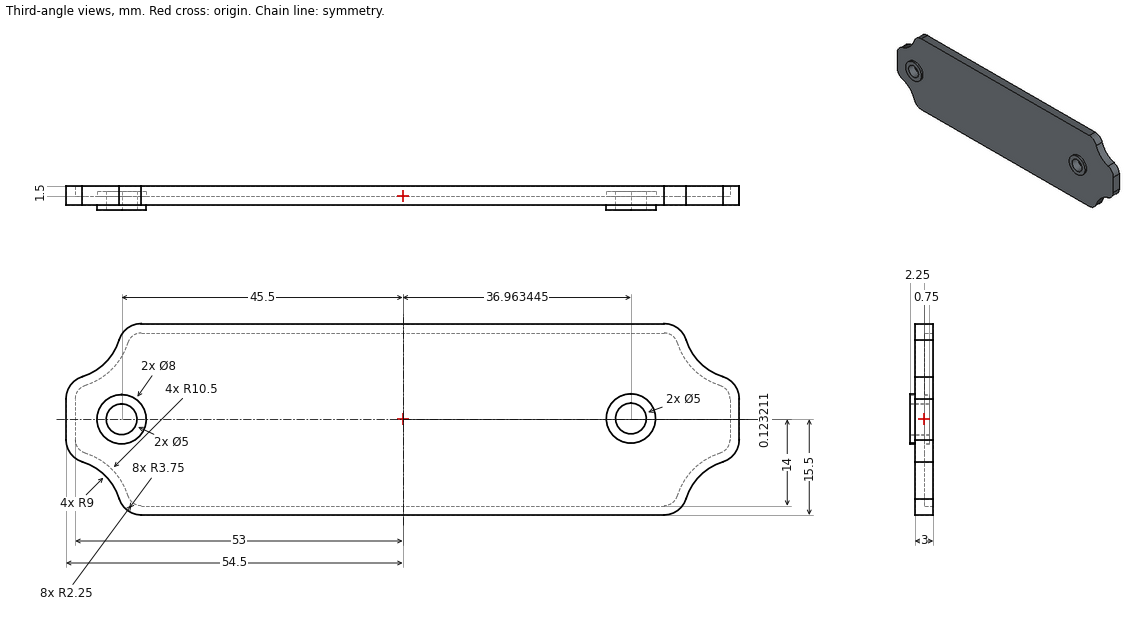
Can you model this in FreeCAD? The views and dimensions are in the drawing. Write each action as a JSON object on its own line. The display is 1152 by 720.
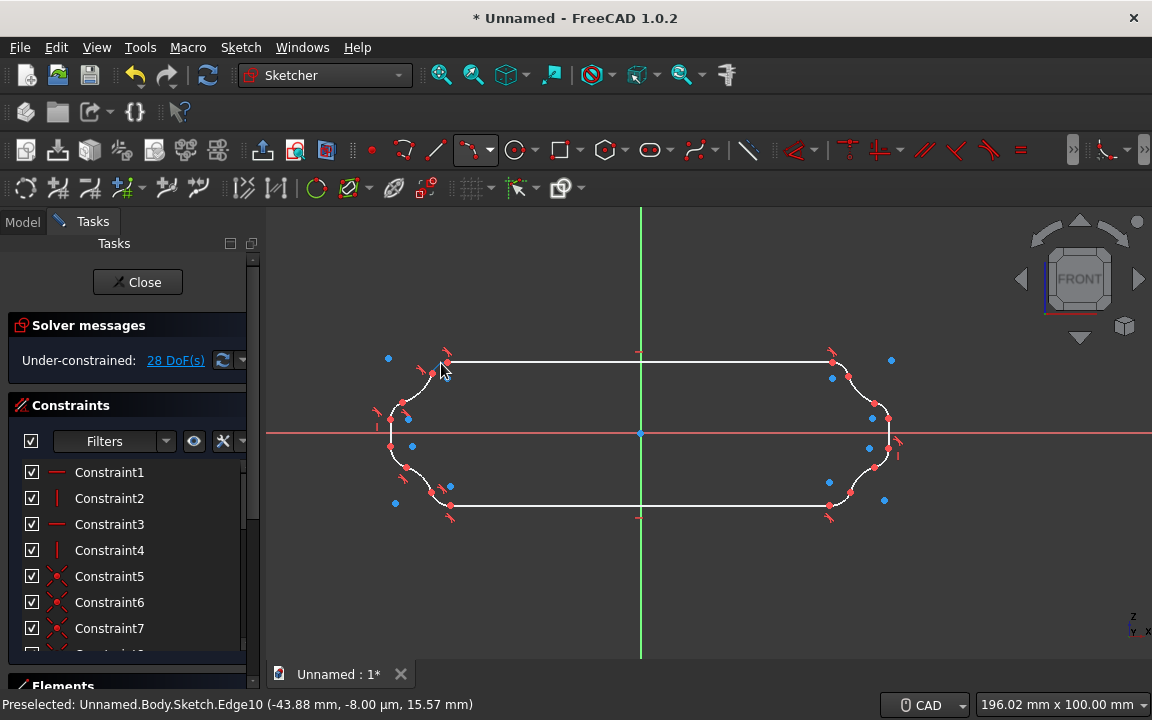
{"action": "scroll", "coordinate": [846, 370], "scroll_direction": "up", "scroll_amount": 4}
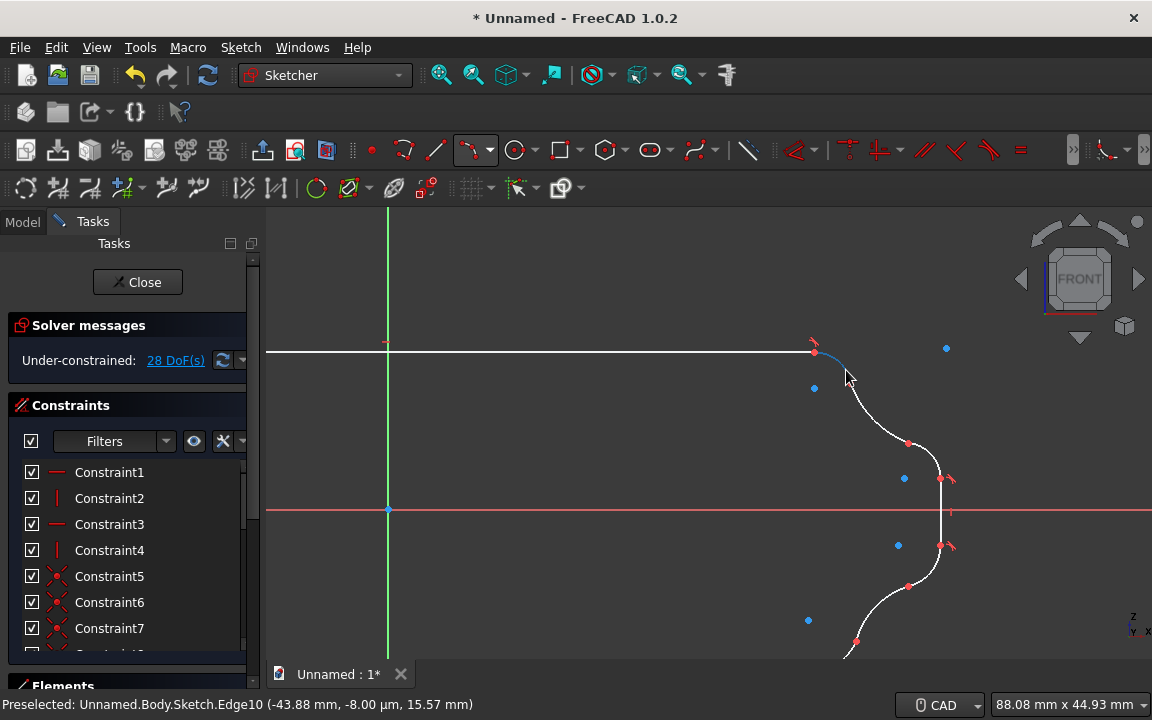
{"action": "left_click", "coordinate": [845, 369]}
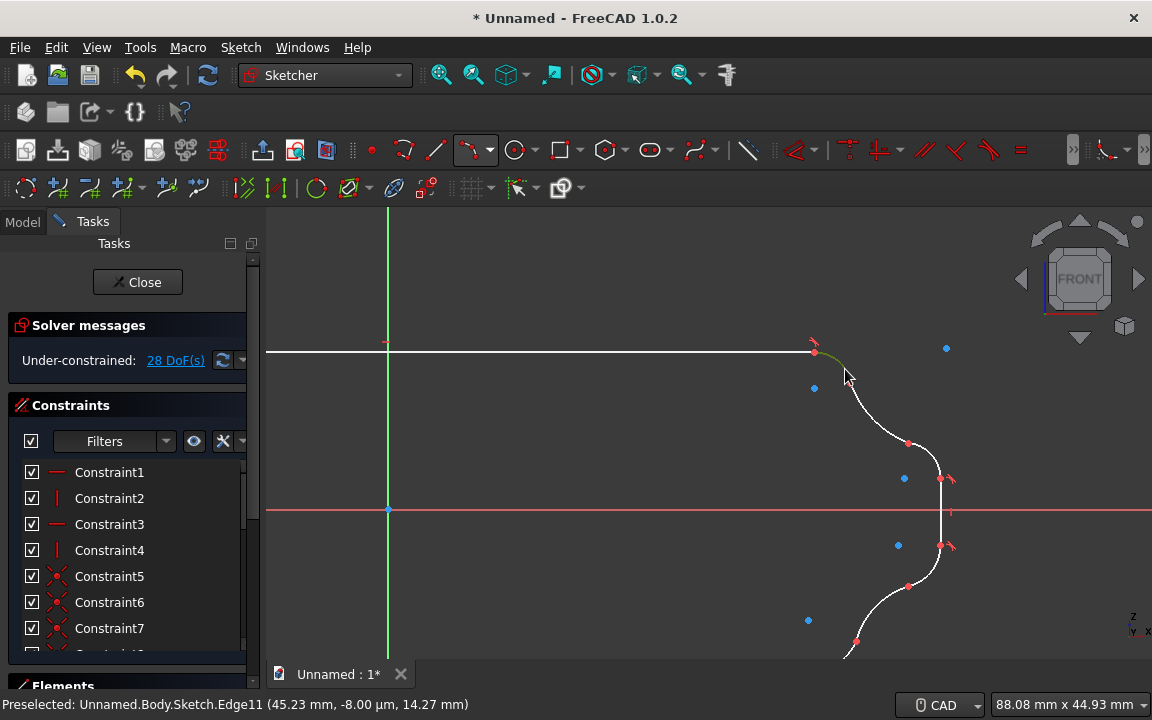
{"action": "left_click", "coordinate": [862, 406]}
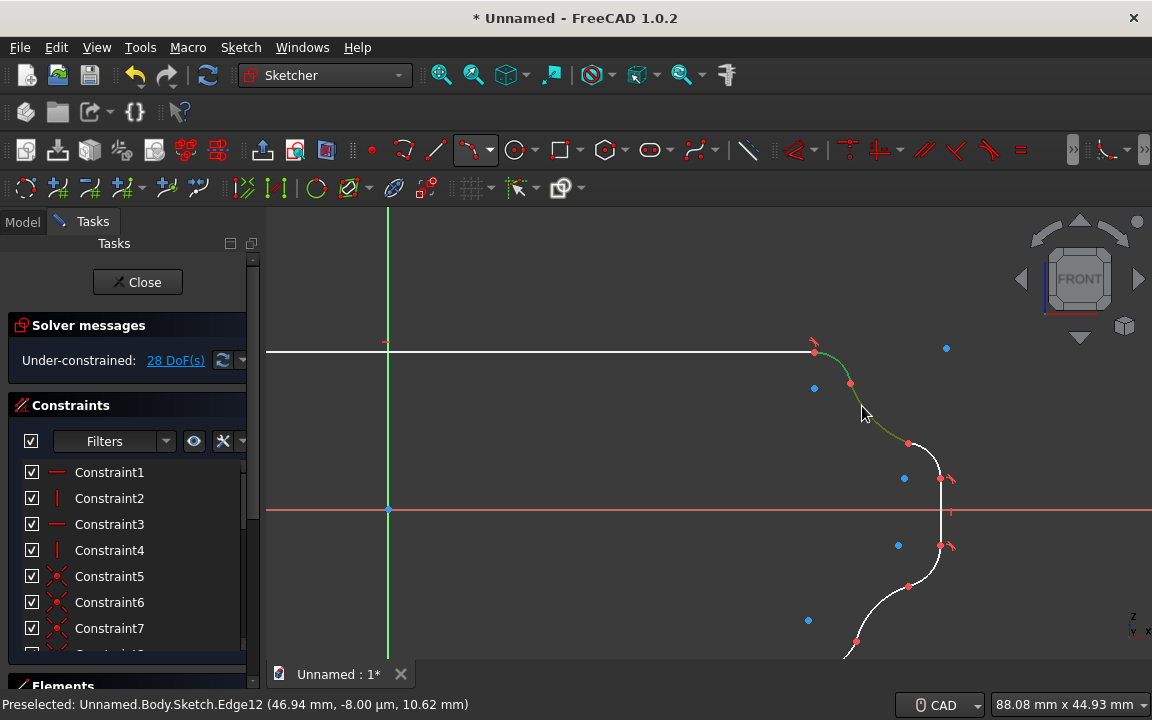
{"action": "left_click", "coordinate": [990, 150]}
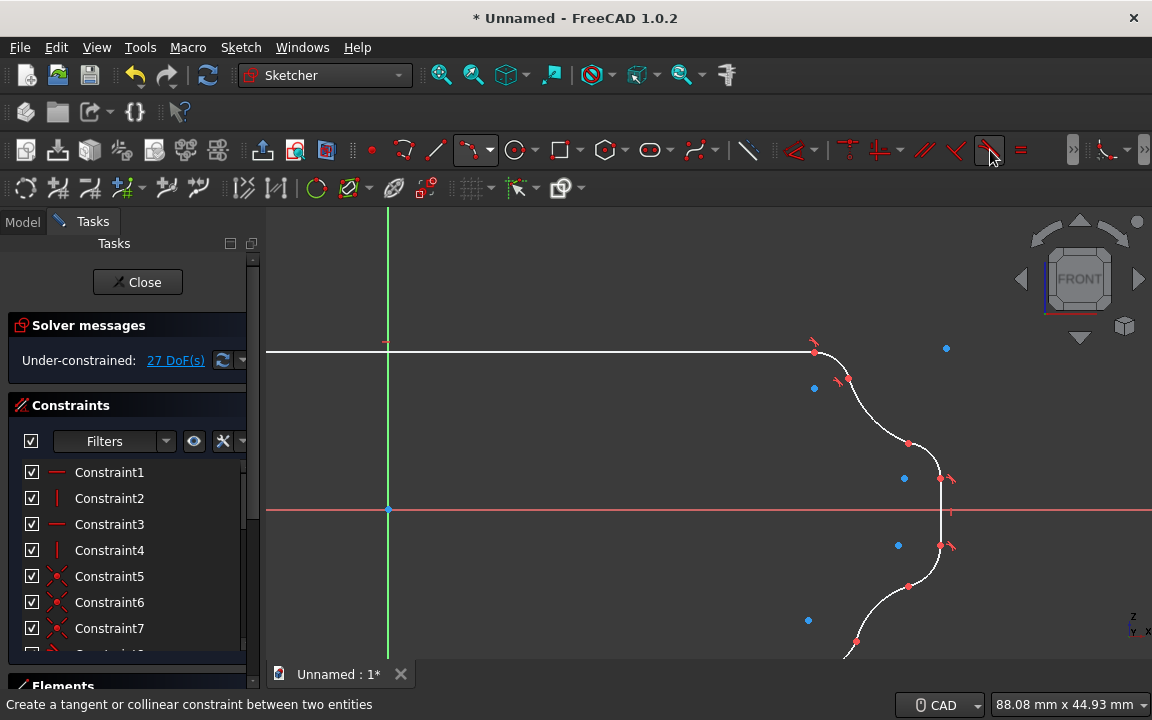
{"action": "left_click", "coordinate": [860, 403]}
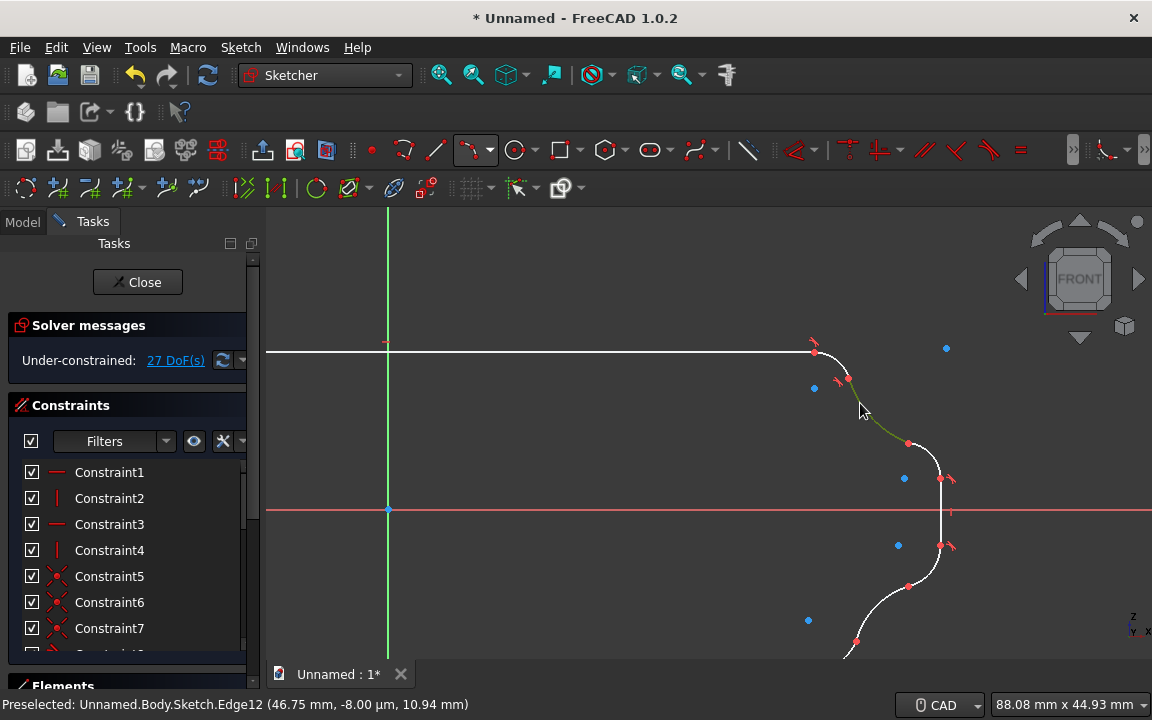
{"action": "left_click", "coordinate": [937, 463]}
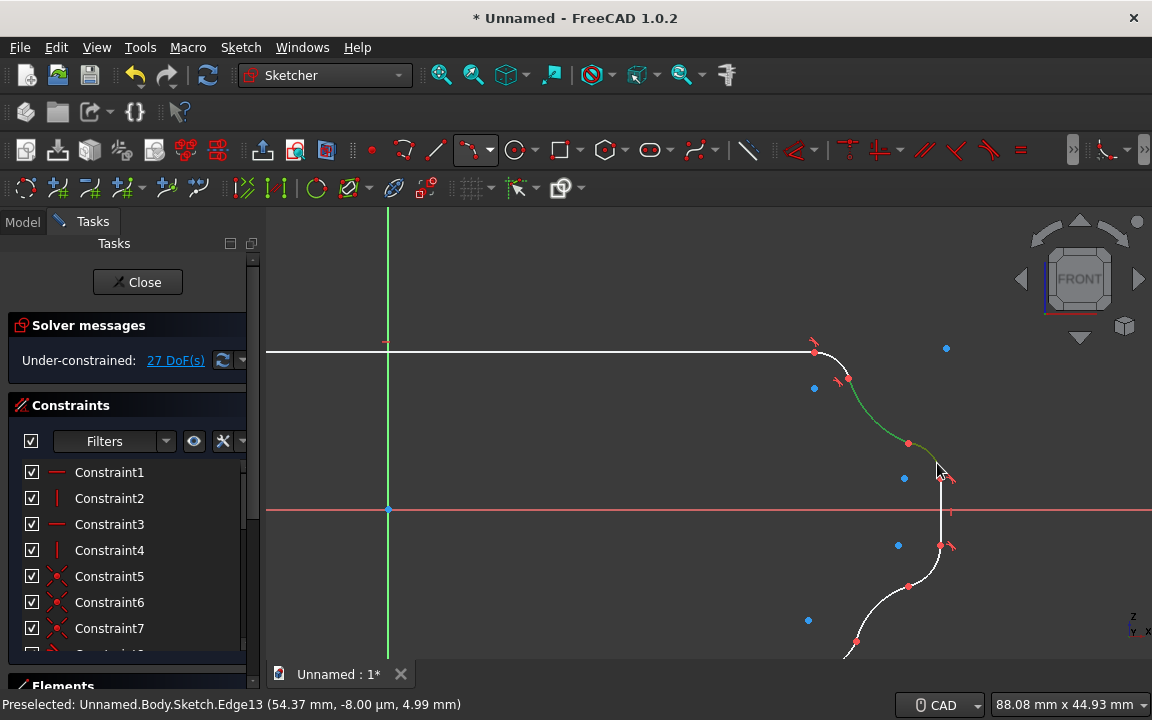
{"action": "left_click", "coordinate": [990, 150]}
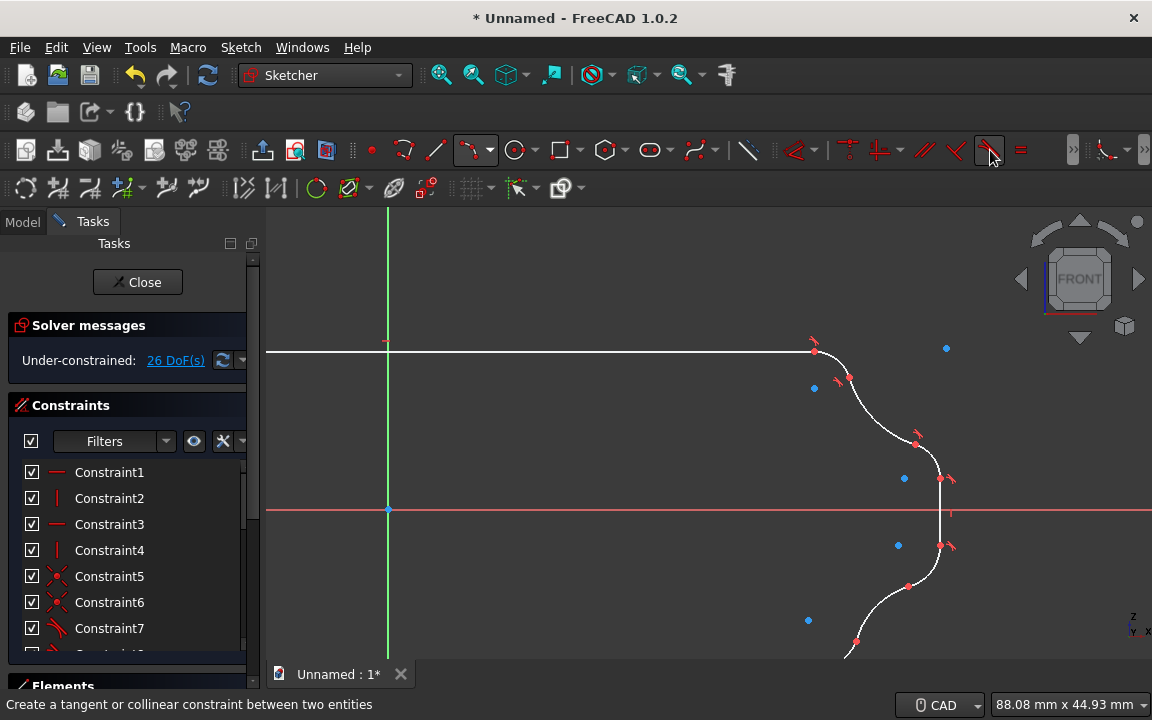
{"action": "left_click", "coordinate": [924, 579]}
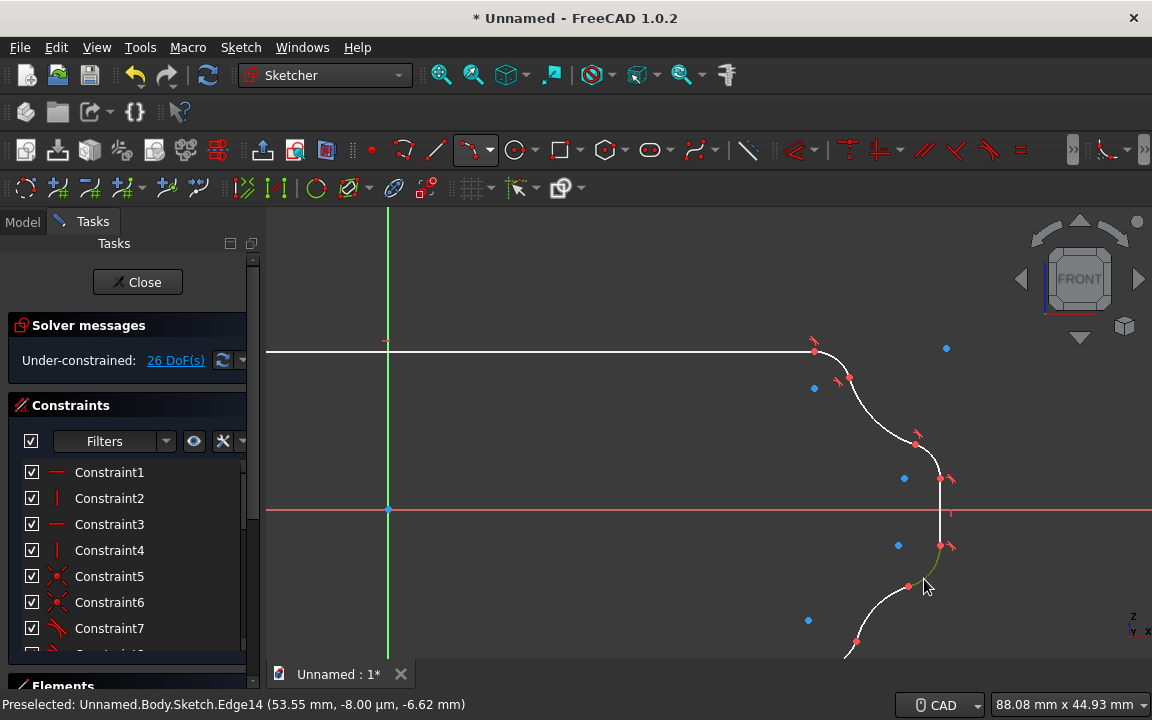
{"action": "left_click", "coordinate": [887, 597]}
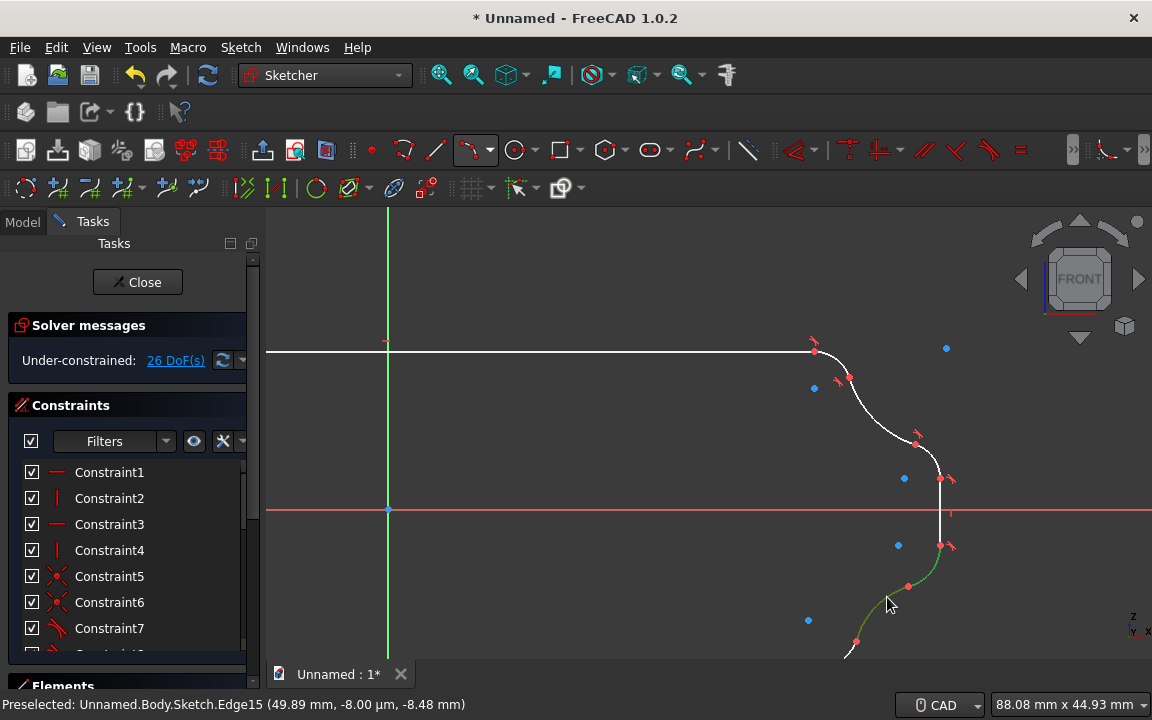
{"action": "left_click", "coordinate": [990, 150]}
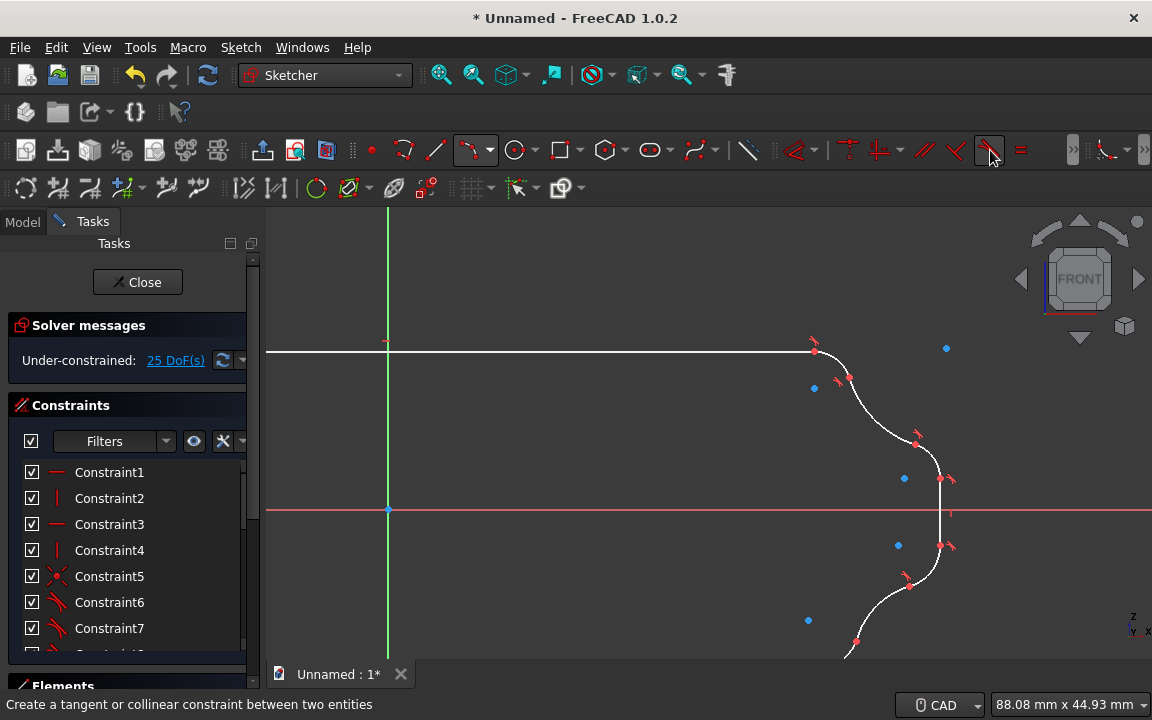
{"action": "left_click", "coordinate": [888, 597]}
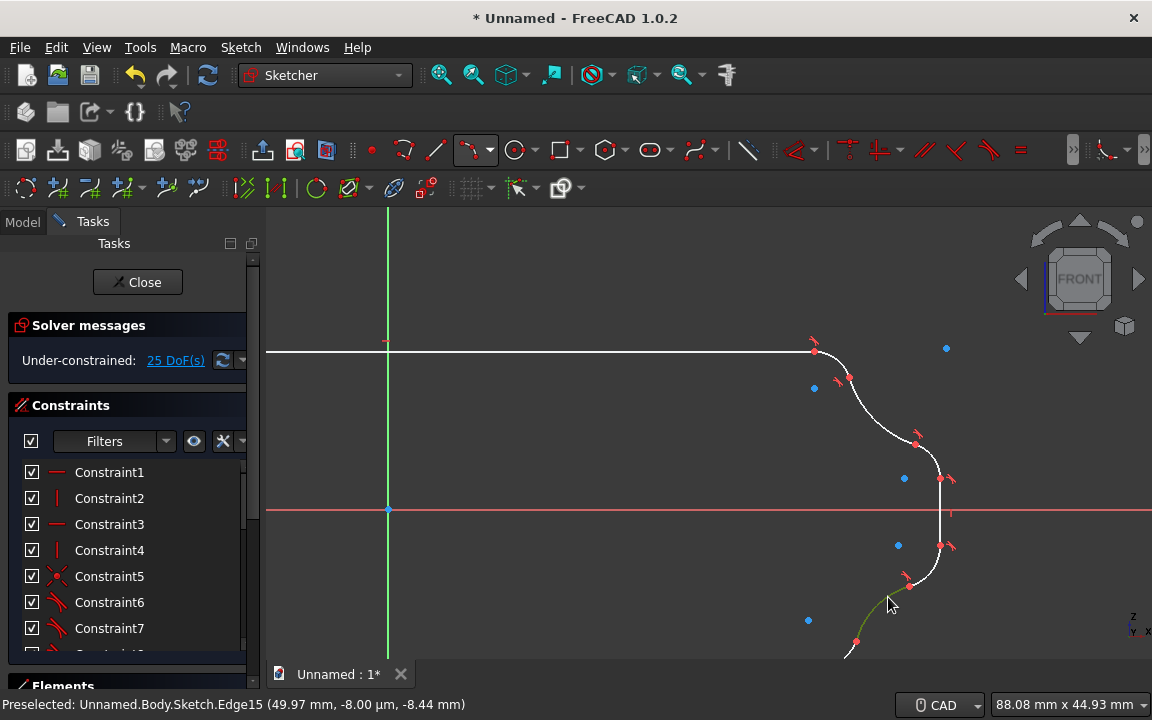
{"action": "scroll", "coordinate": [846, 370], "scroll_direction": "down", "scroll_amount": 4}